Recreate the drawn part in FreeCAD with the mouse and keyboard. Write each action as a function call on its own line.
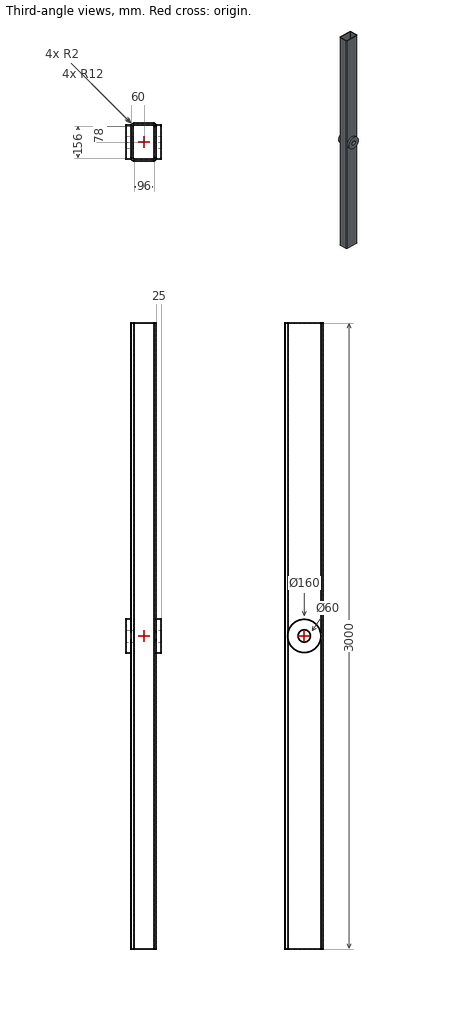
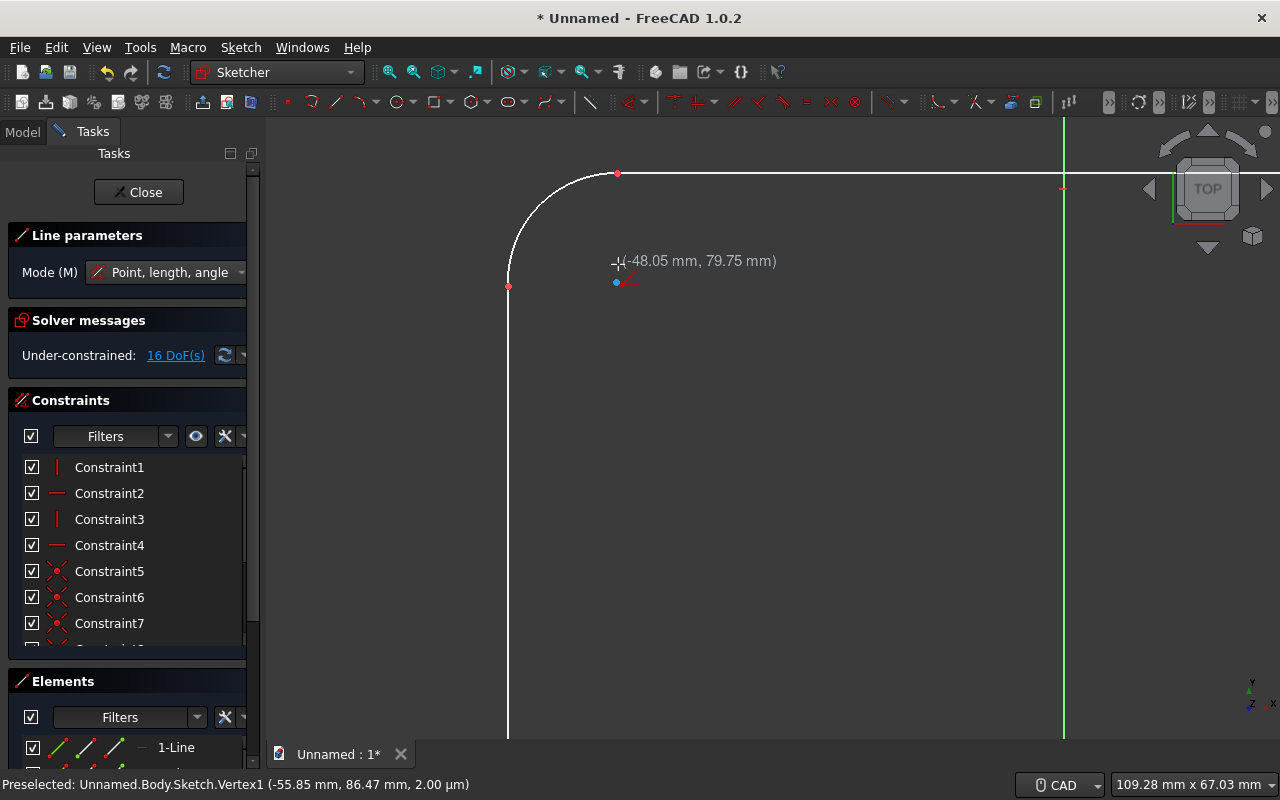
click(618, 263)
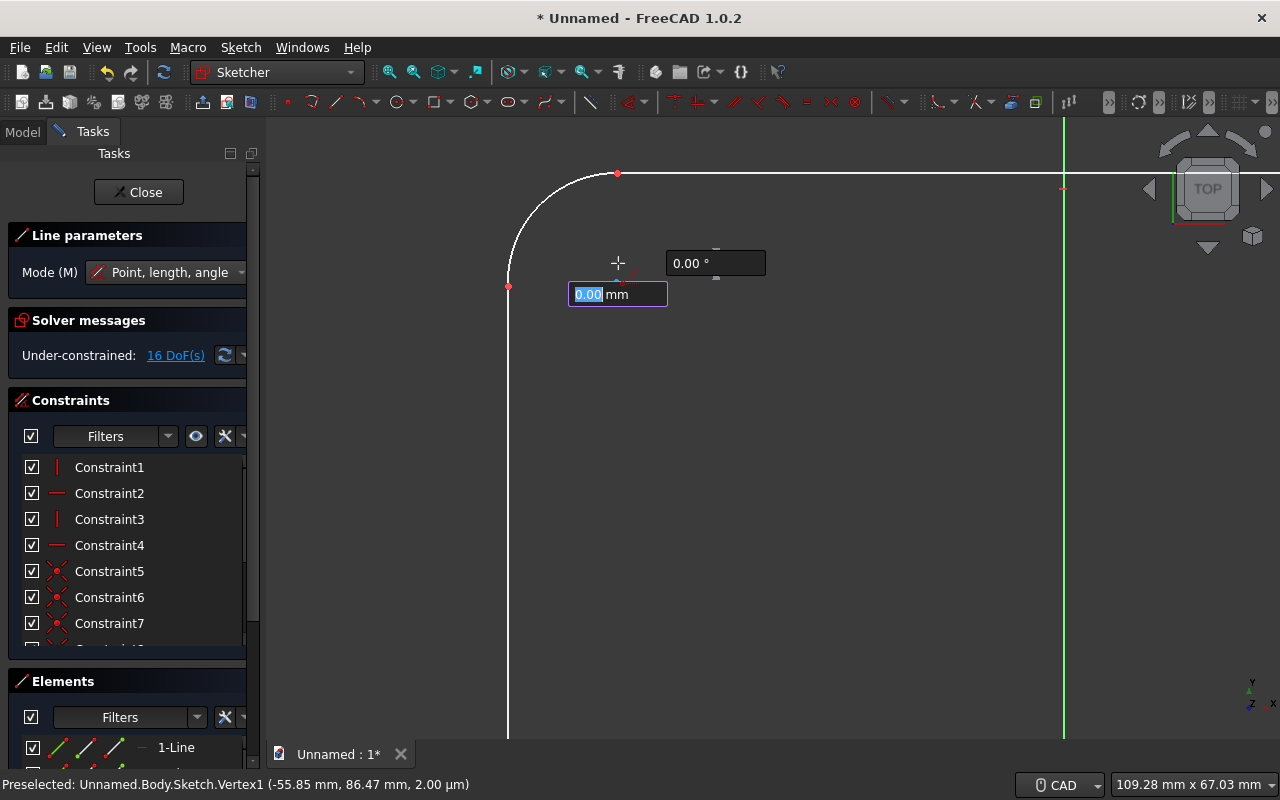
scroll(587, 239, down, 7)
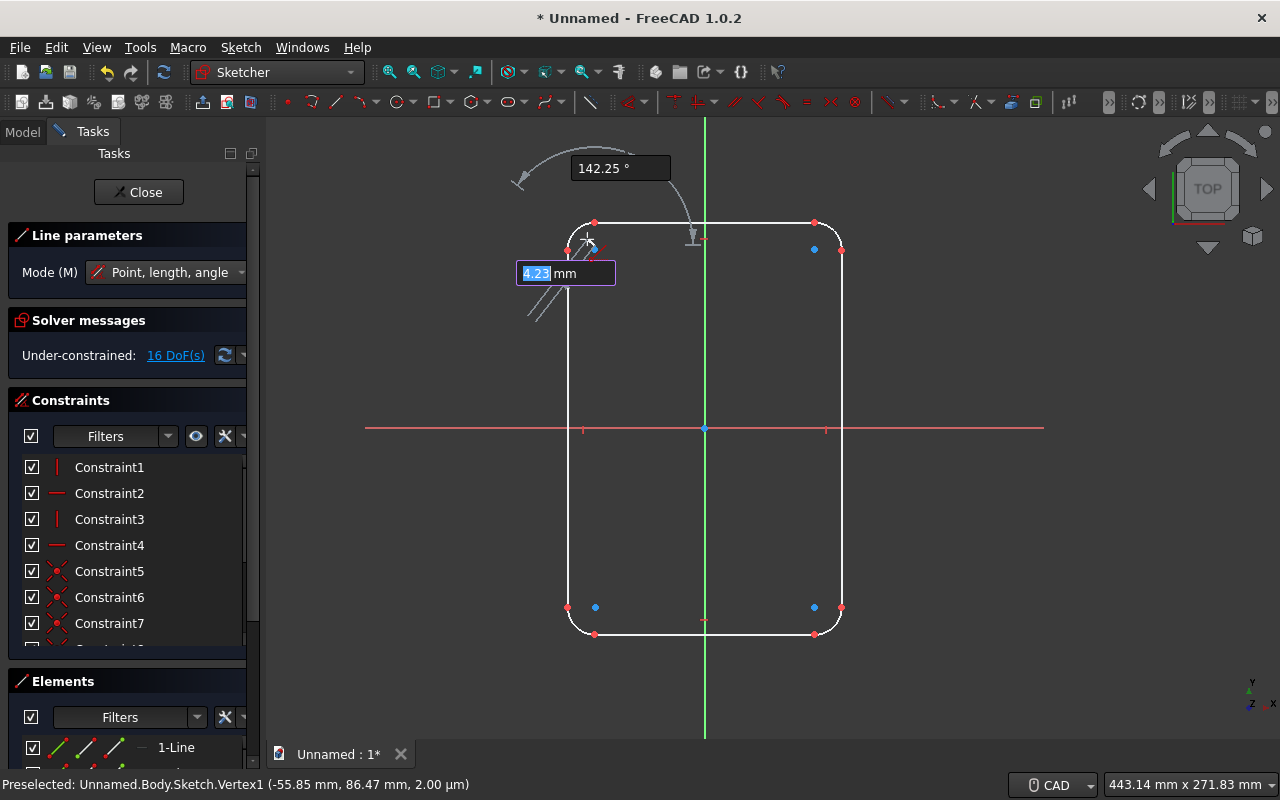
scroll(815, 245, up, 7)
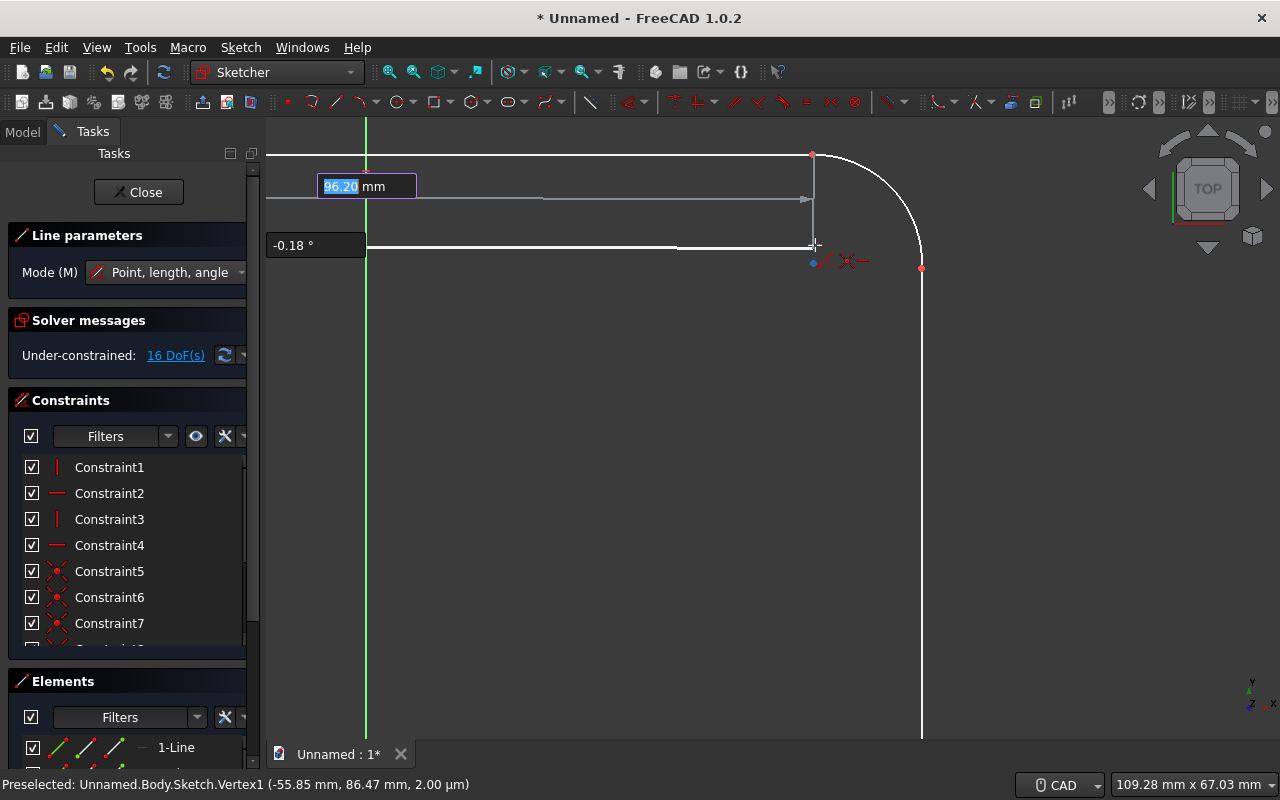
click(812, 245)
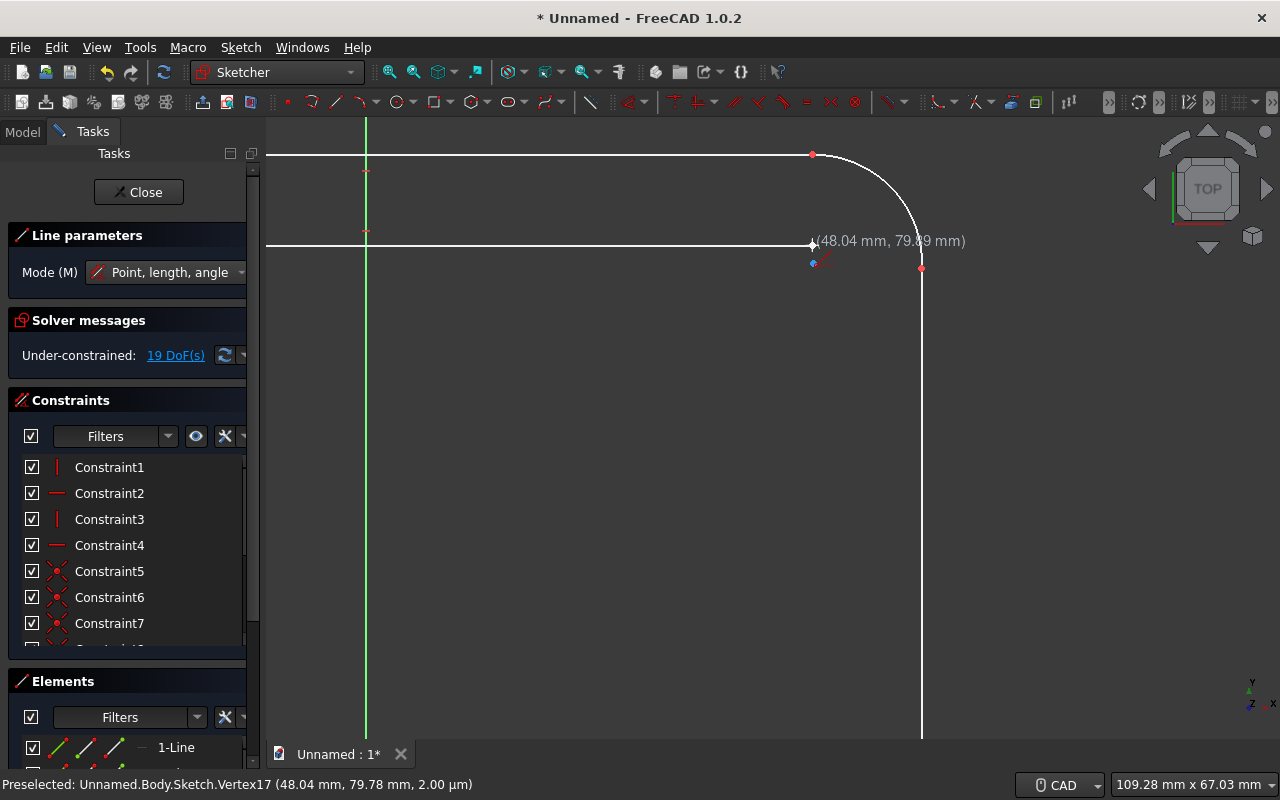
click(830, 264)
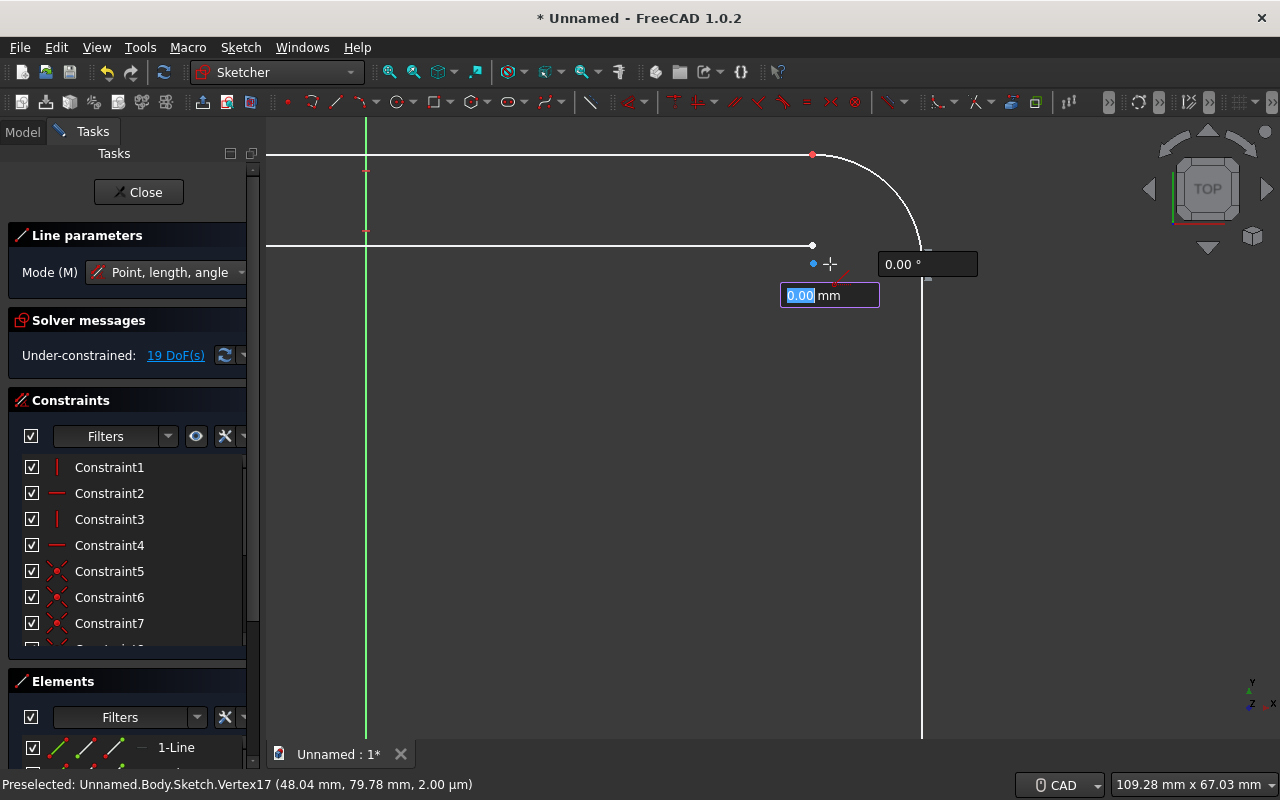
scroll(815, 245, down, 7)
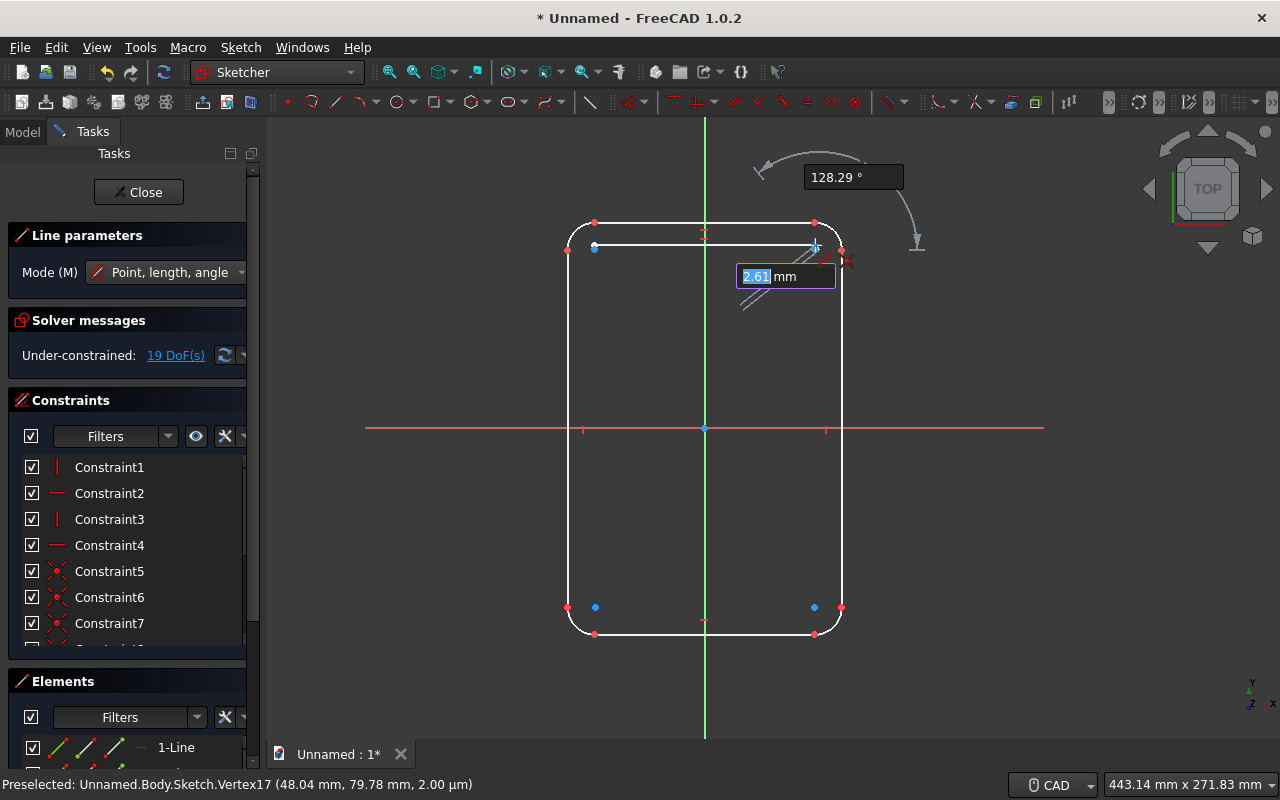
scroll(819, 607, up, 7)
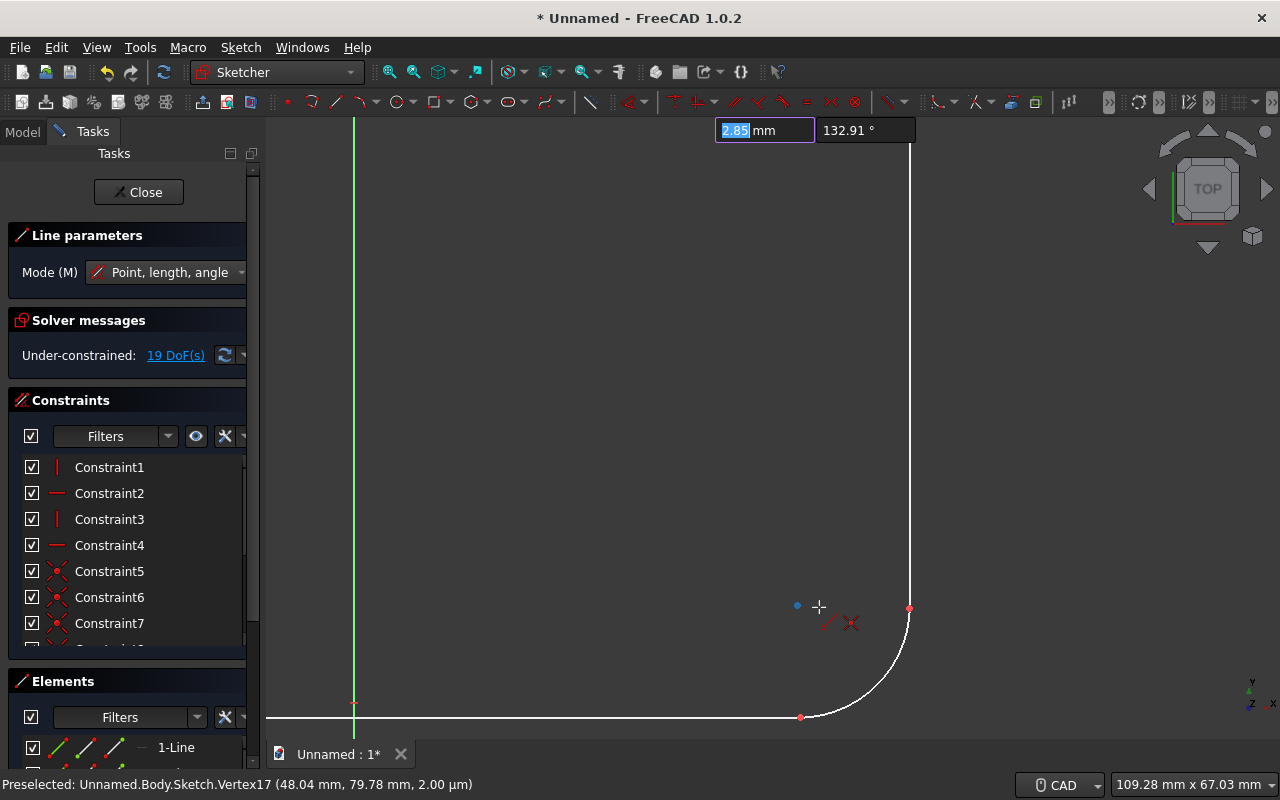
click(818, 603)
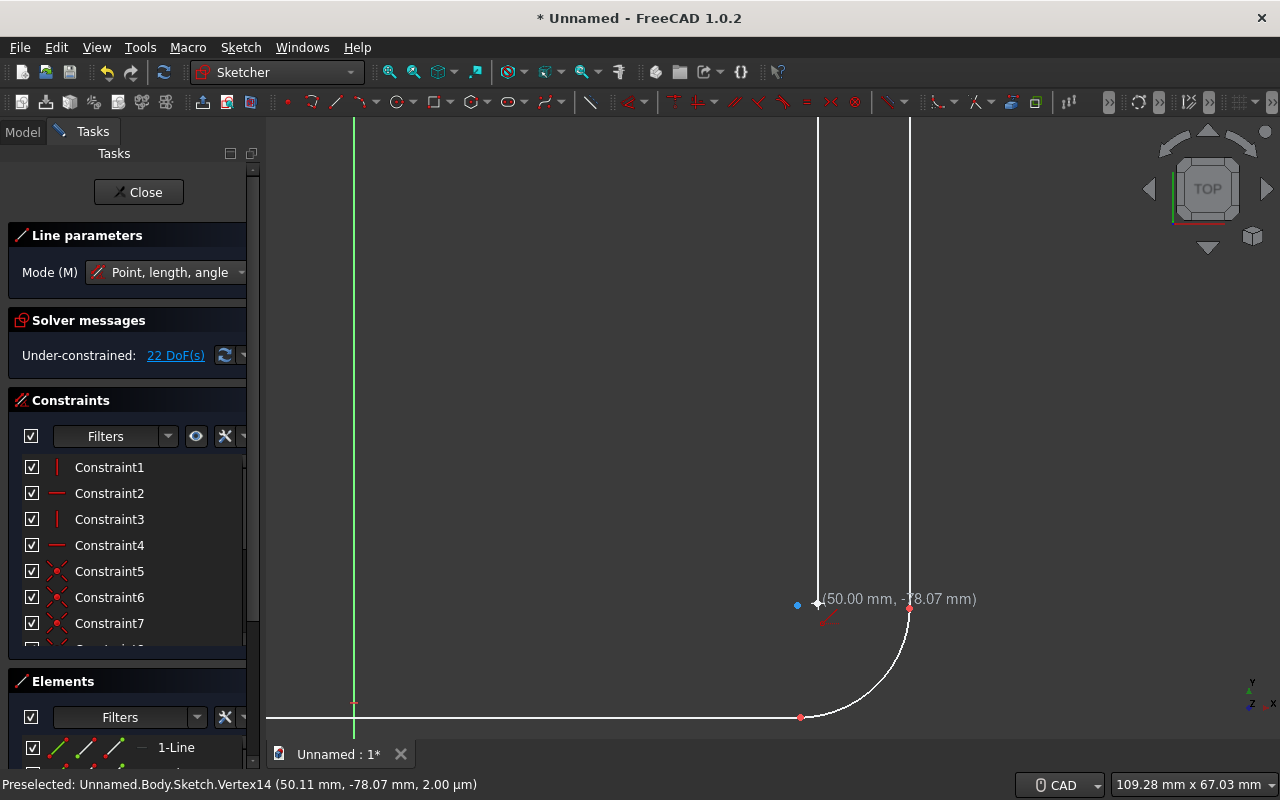
click(799, 622)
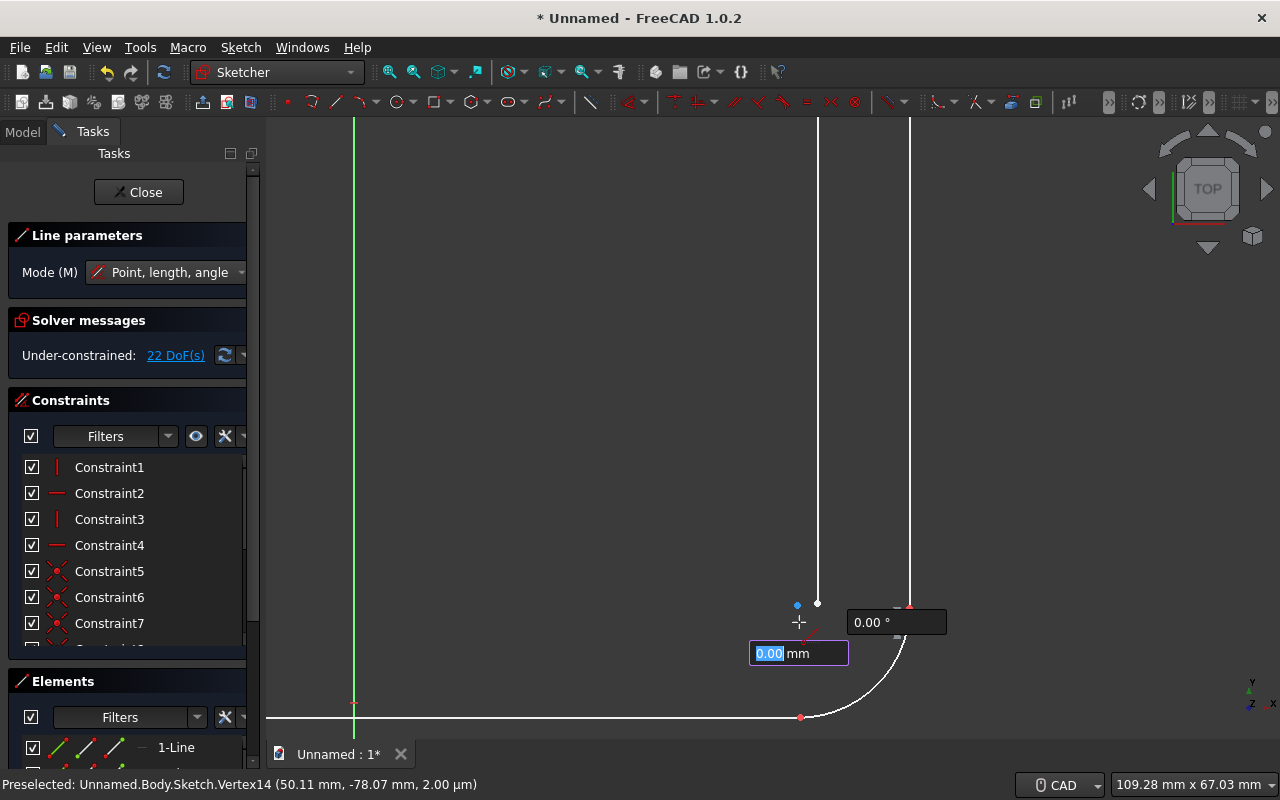
scroll(819, 608, down, 7)